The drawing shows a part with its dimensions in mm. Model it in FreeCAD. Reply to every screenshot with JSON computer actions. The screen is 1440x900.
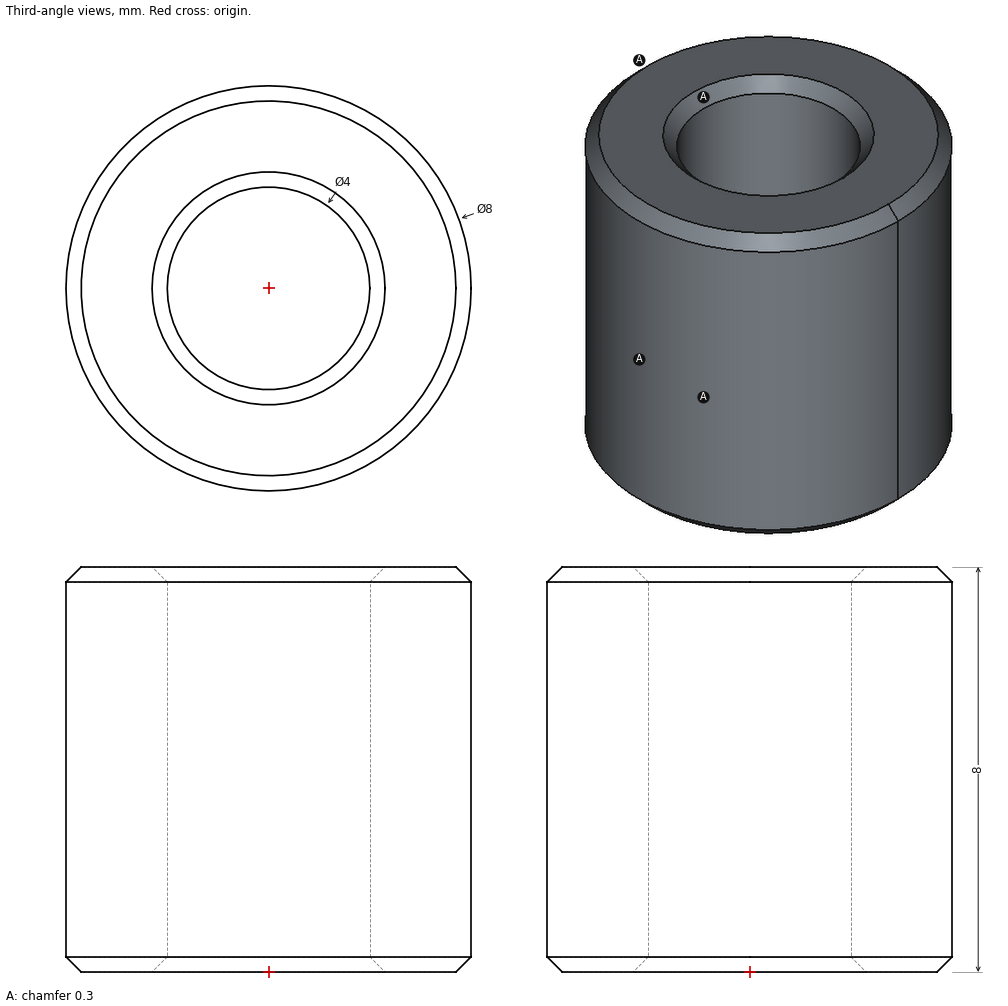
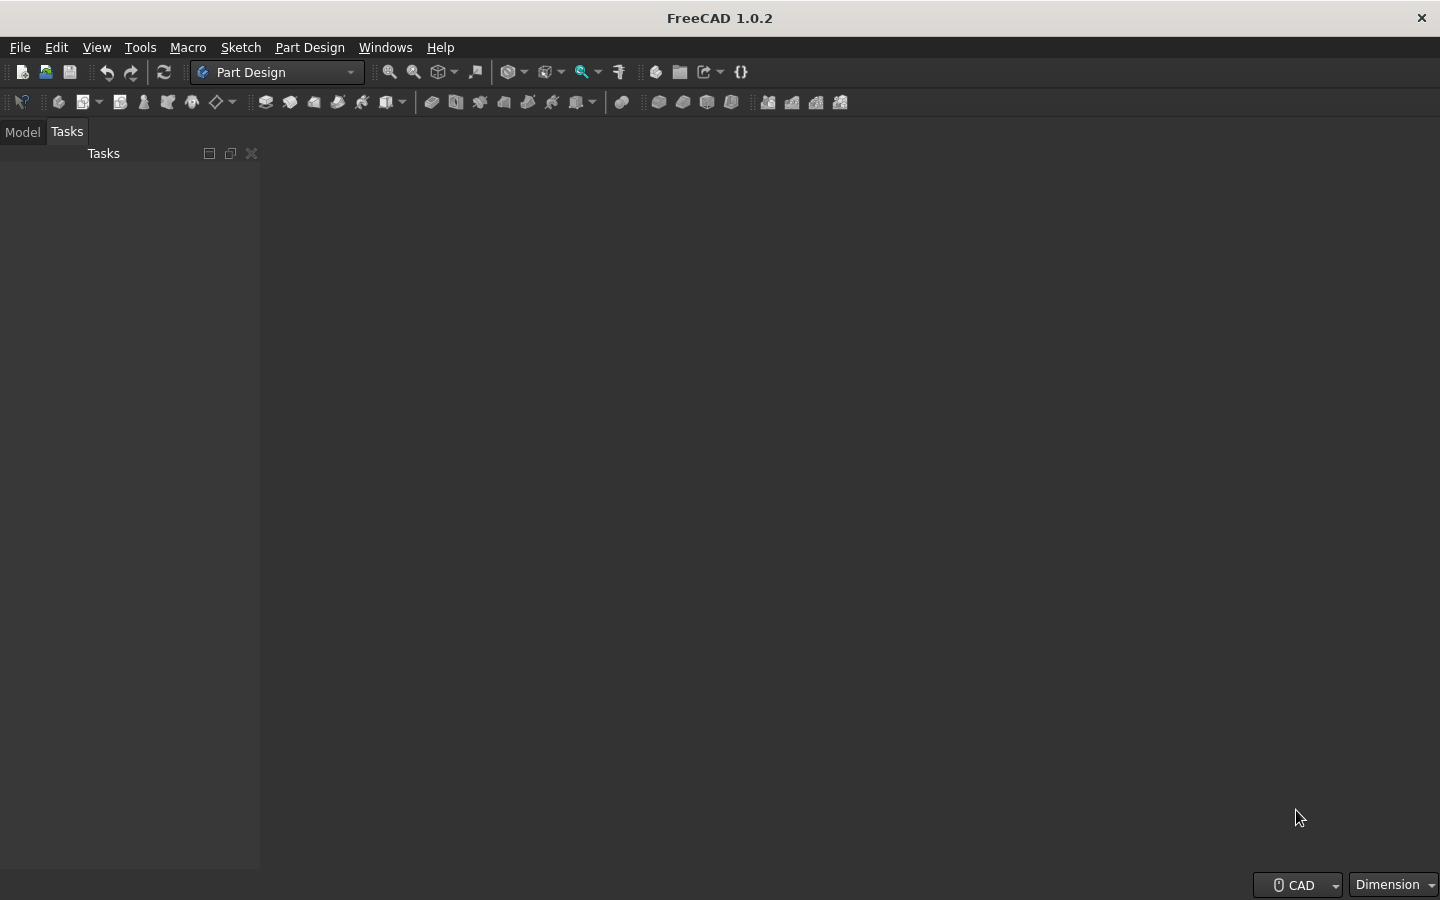
{"action": "left_click", "coordinate": [22, 72]}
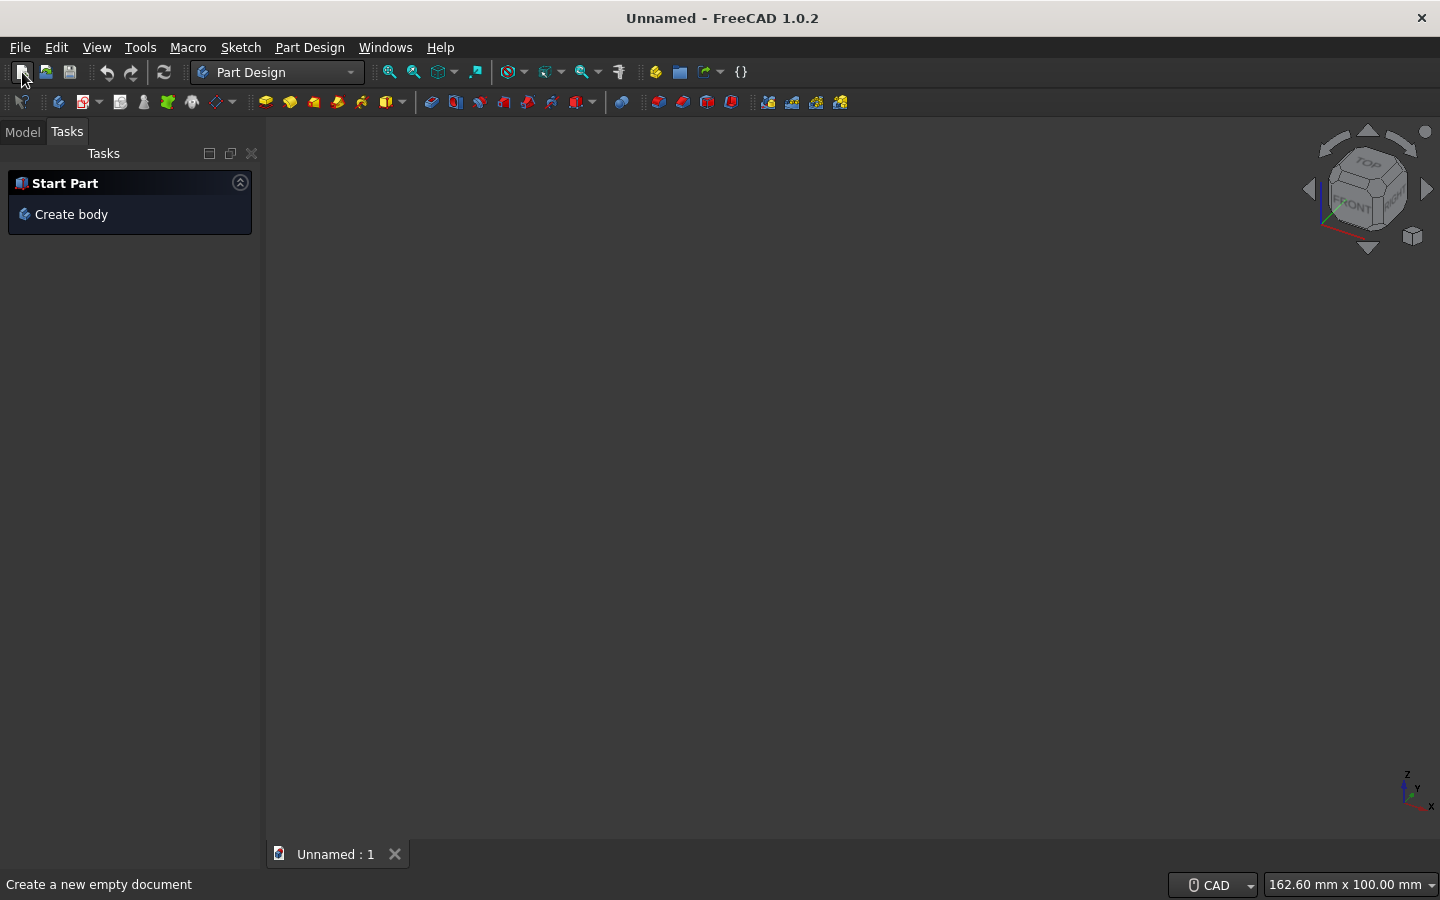
{"action": "left_click", "coordinate": [84, 102]}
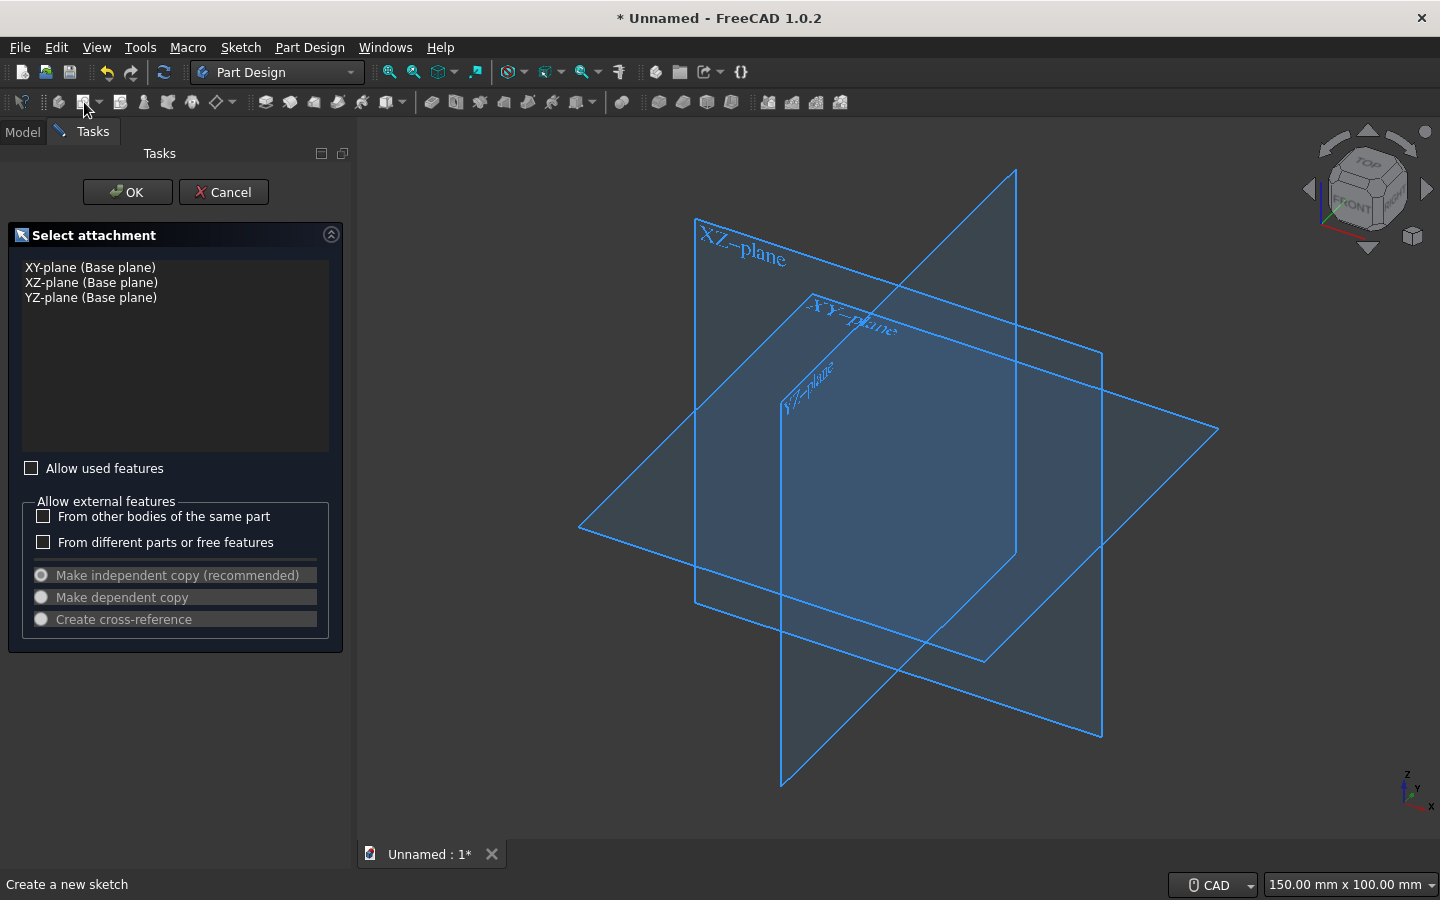
{"action": "left_click", "coordinate": [82, 268]}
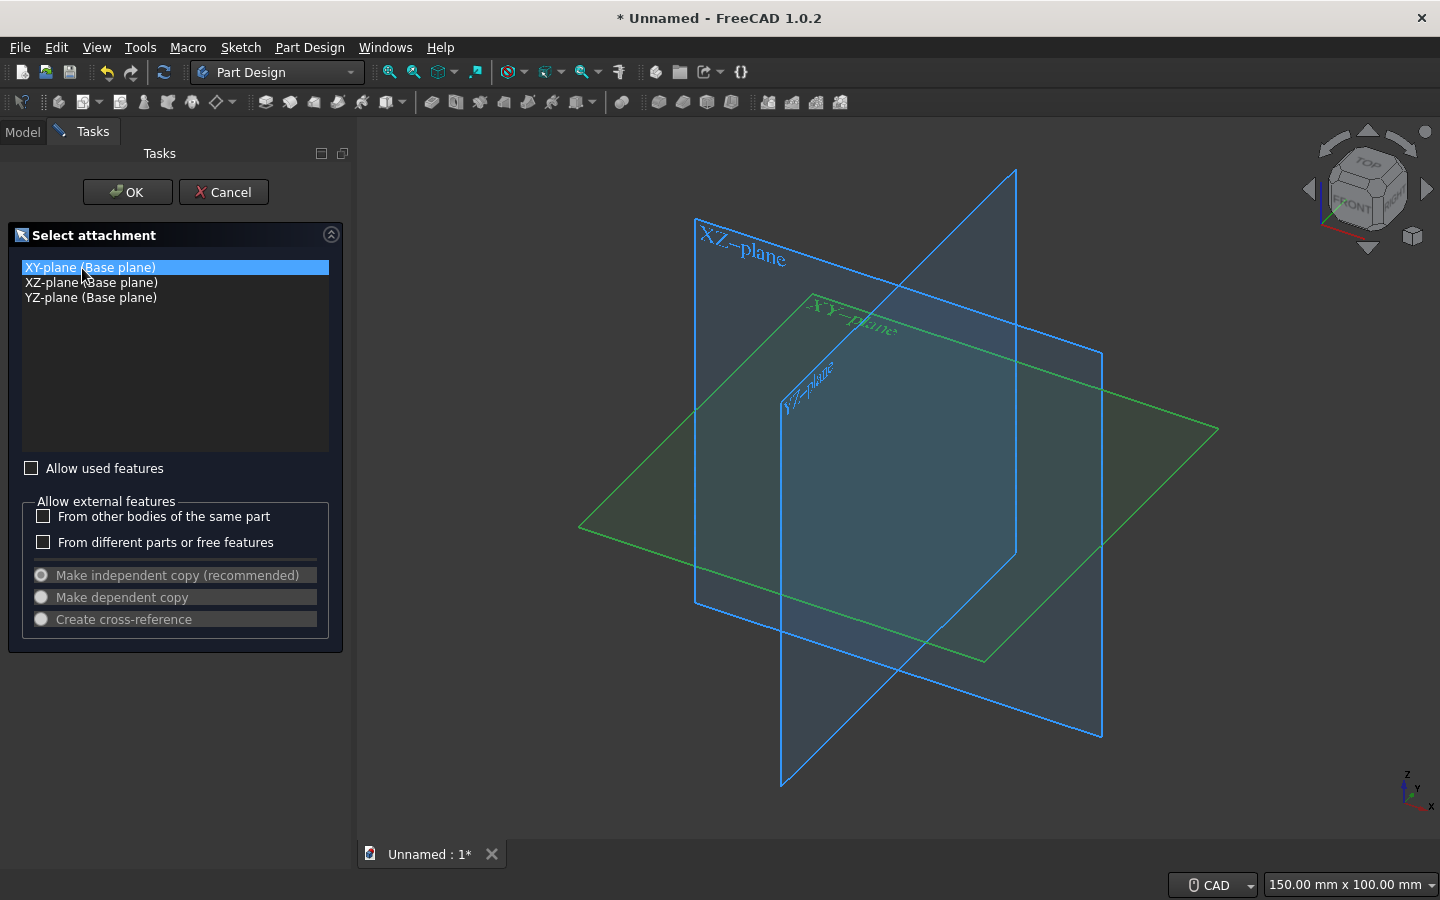
{"action": "left_click", "coordinate": [128, 192]}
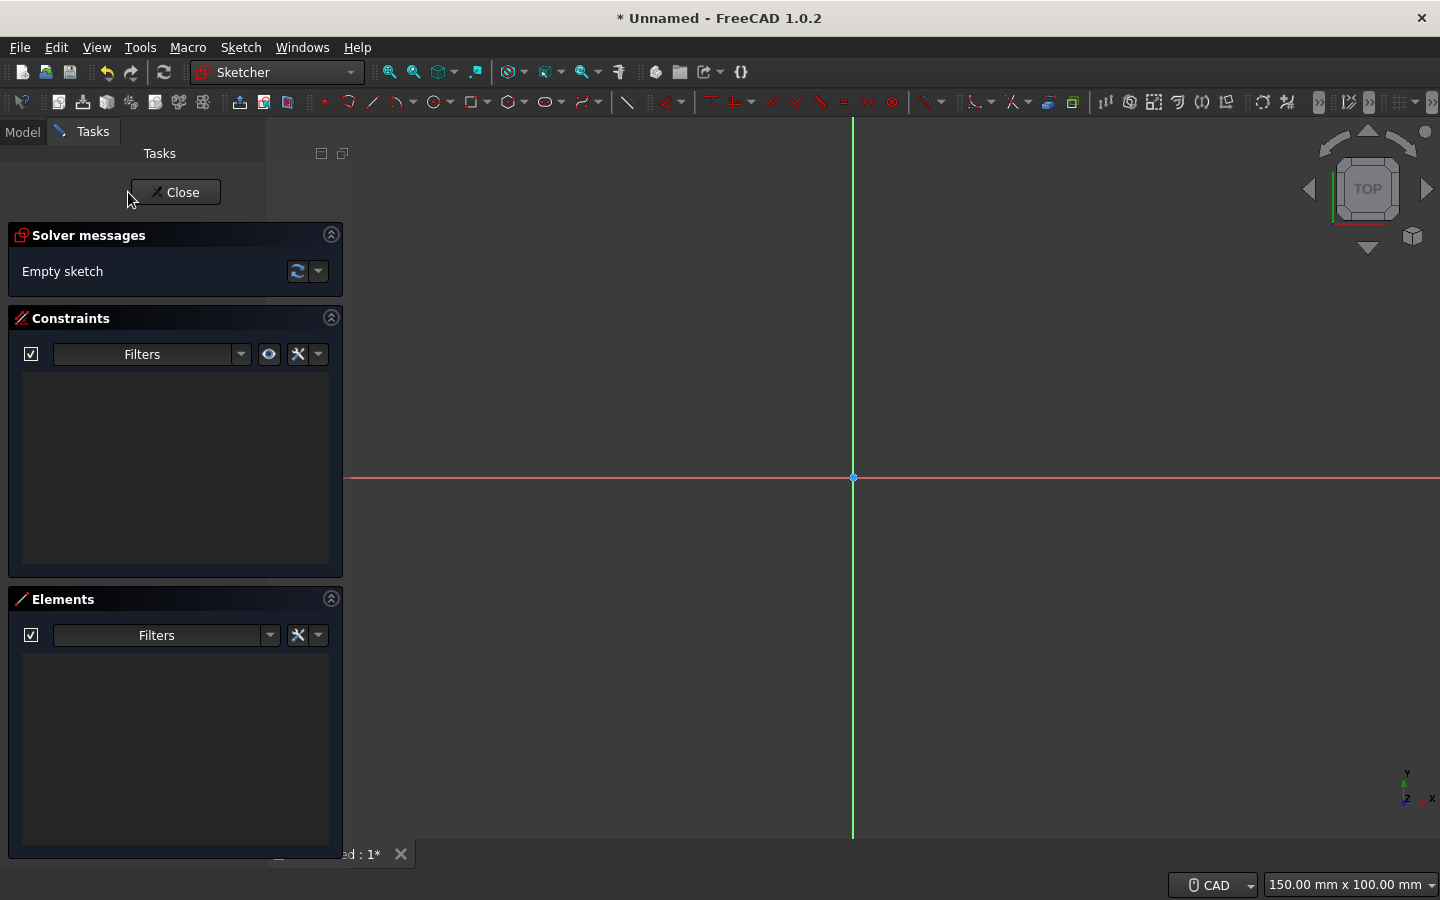
{"action": "scroll", "coordinate": [864, 478], "scroll_direction": "up", "scroll_amount": 10}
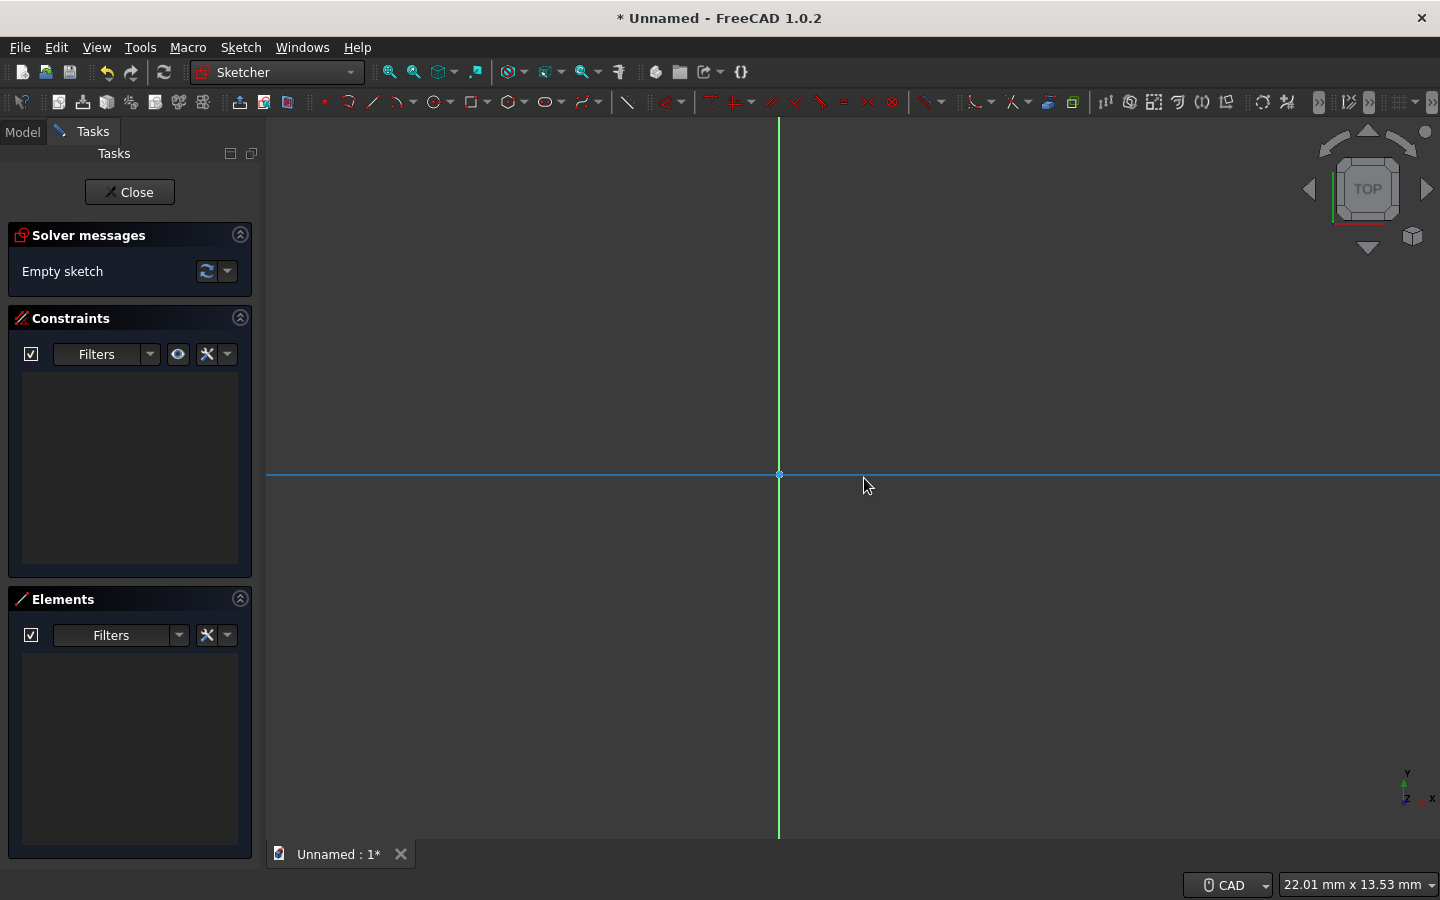
{"action": "key", "text": "g c"}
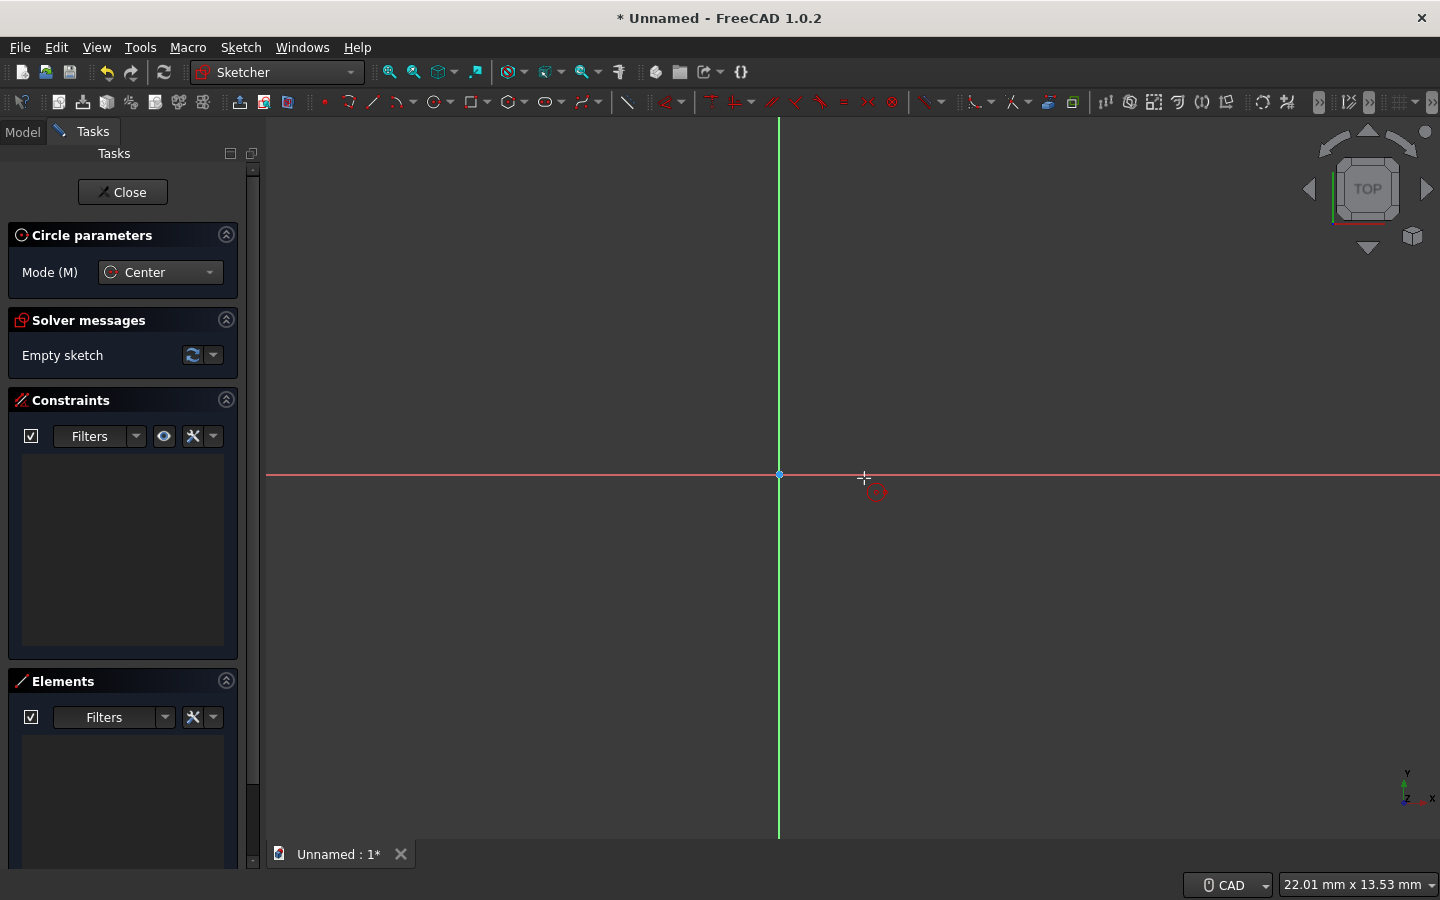
{"action": "left_click", "coordinate": [779, 475]}
{"action": "left_click", "coordinate": [930, 324]}